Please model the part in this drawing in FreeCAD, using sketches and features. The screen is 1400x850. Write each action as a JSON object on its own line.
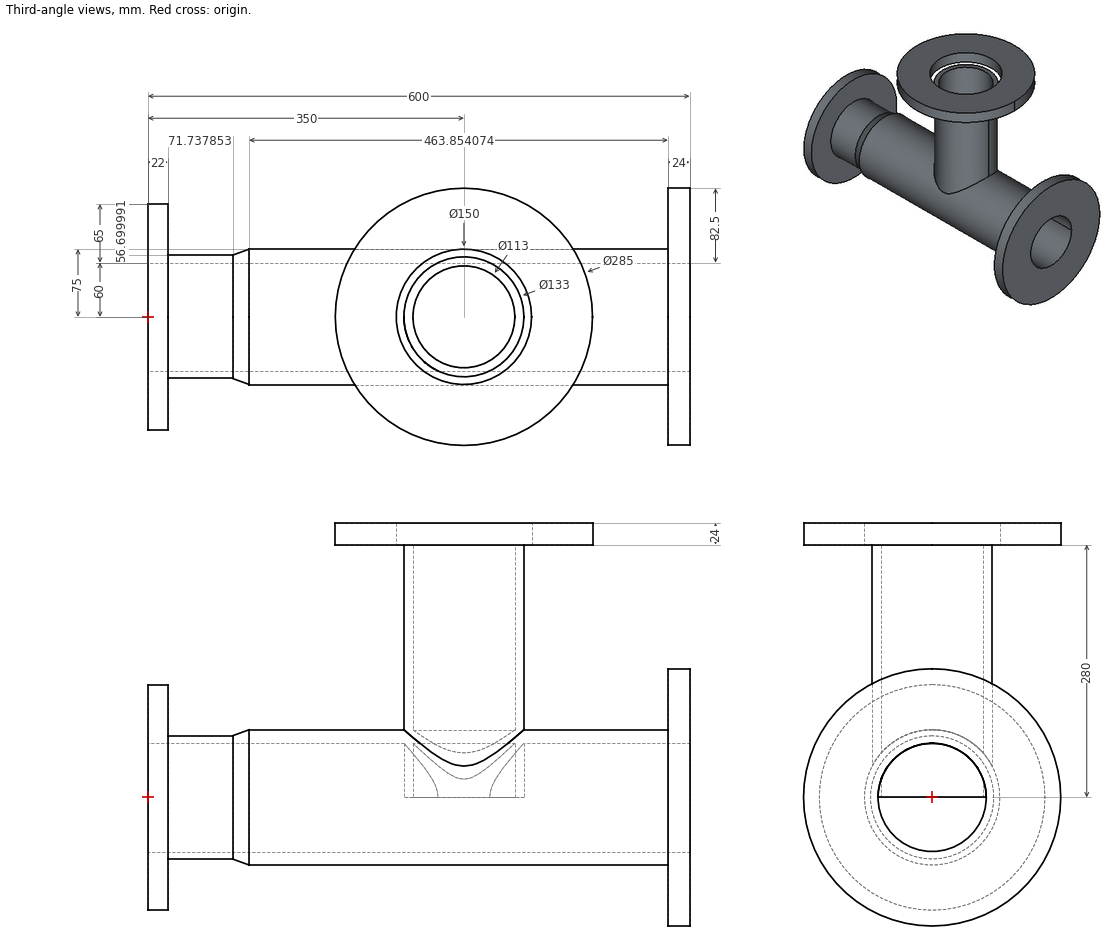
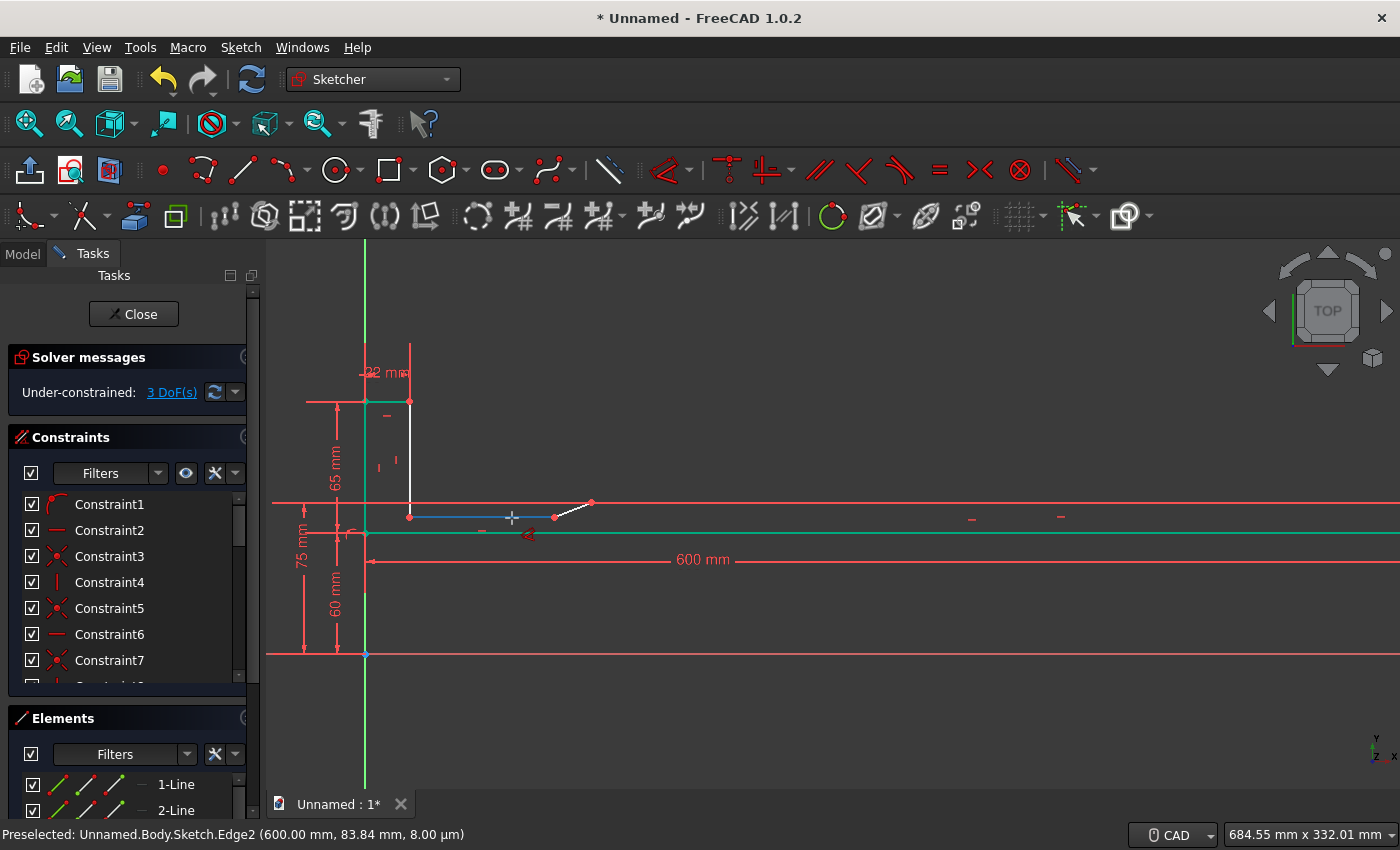
{"action": "left_click", "coordinate": [511, 517]}
{"action": "left_click", "coordinate": [482, 551]}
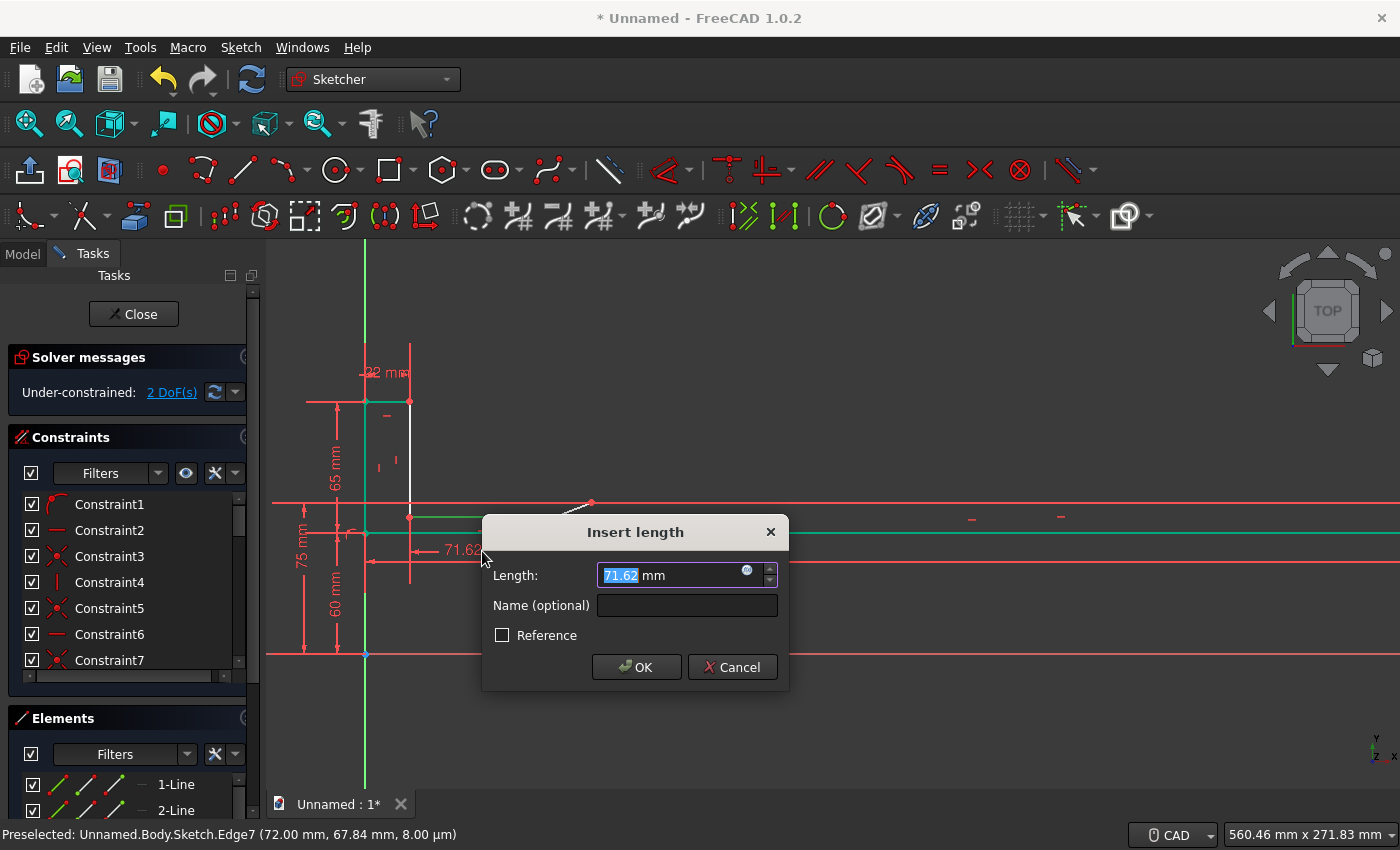
{"action": "type", "text": "71.737853"}
{"action": "key", "text": "Return"}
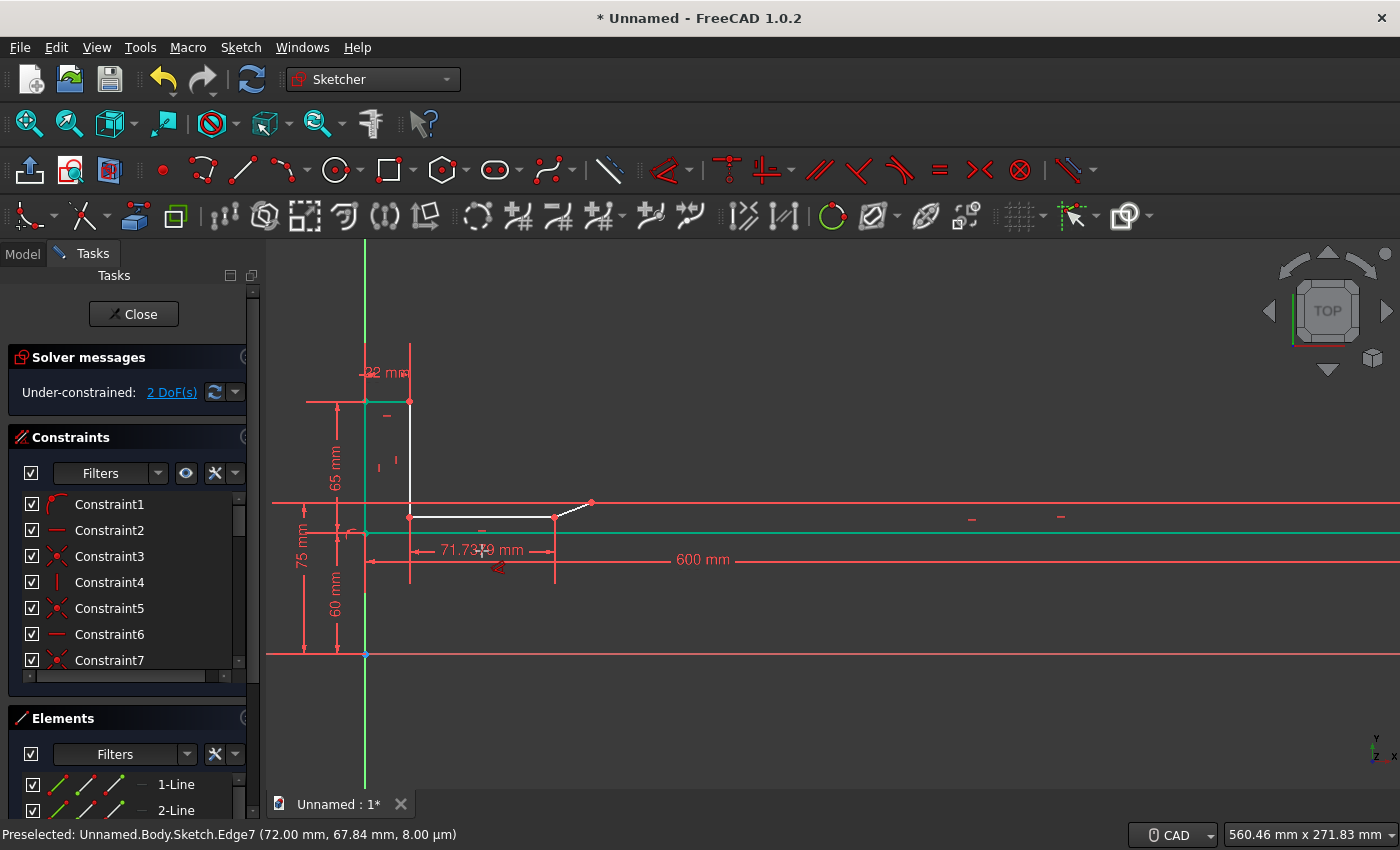
{"action": "left_click", "coordinate": [410, 482]}
{"action": "left_click", "coordinate": [444, 459]}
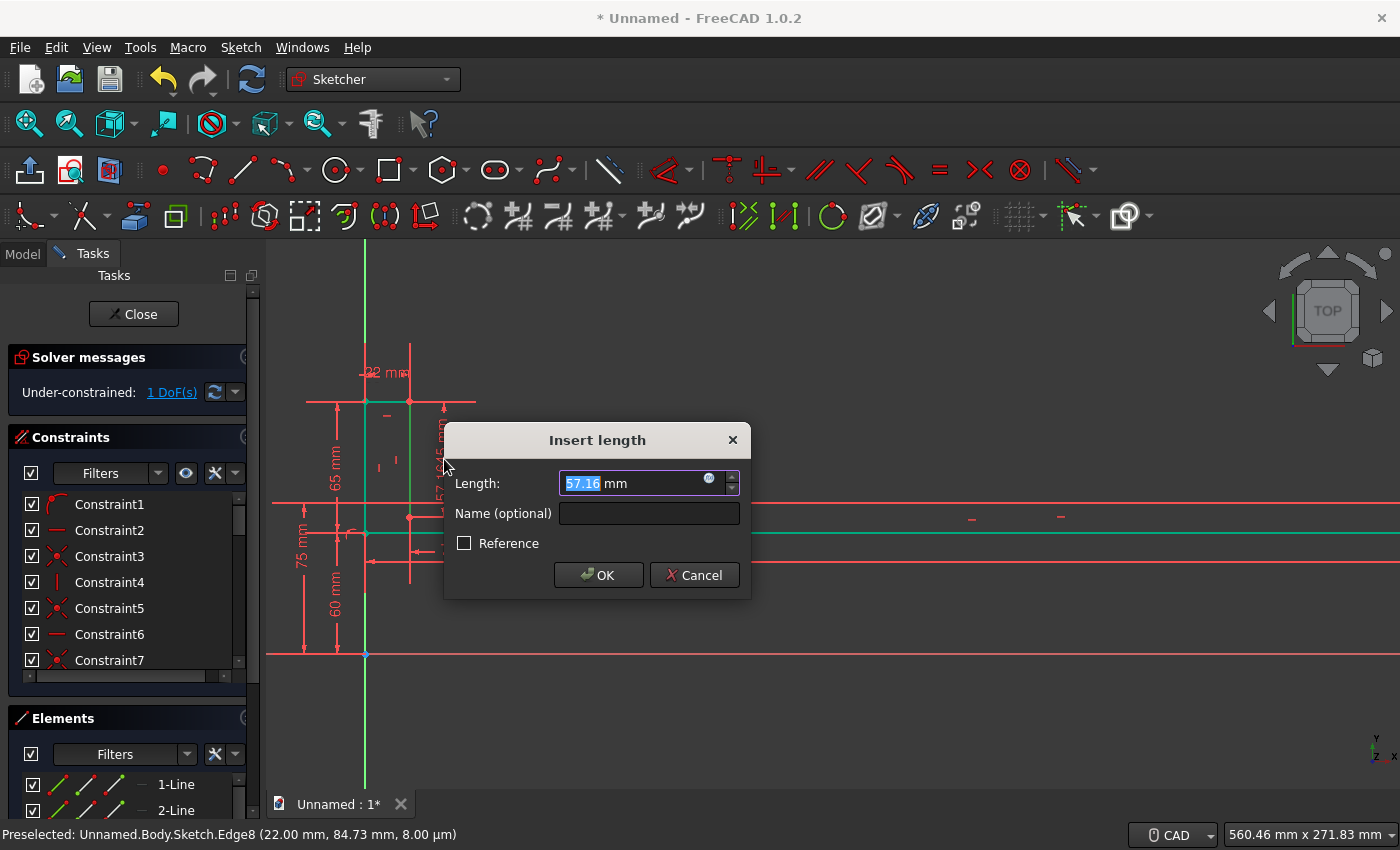
{"action": "type", "text": "56.699991"}
{"action": "key", "text": "Return"}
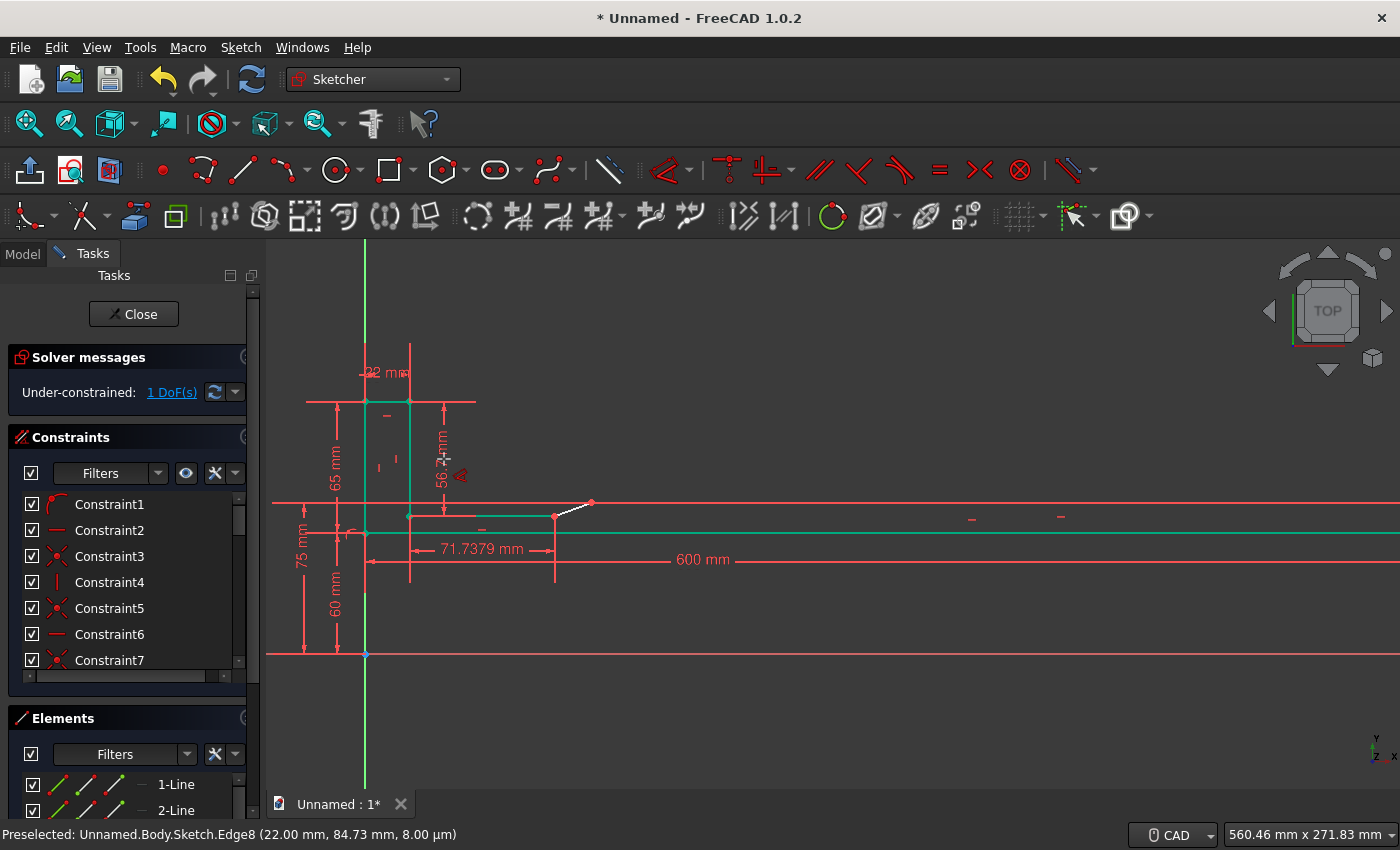
{"action": "left_click", "coordinate": [874, 503]}
{"action": "left_click", "coordinate": [913, 469]}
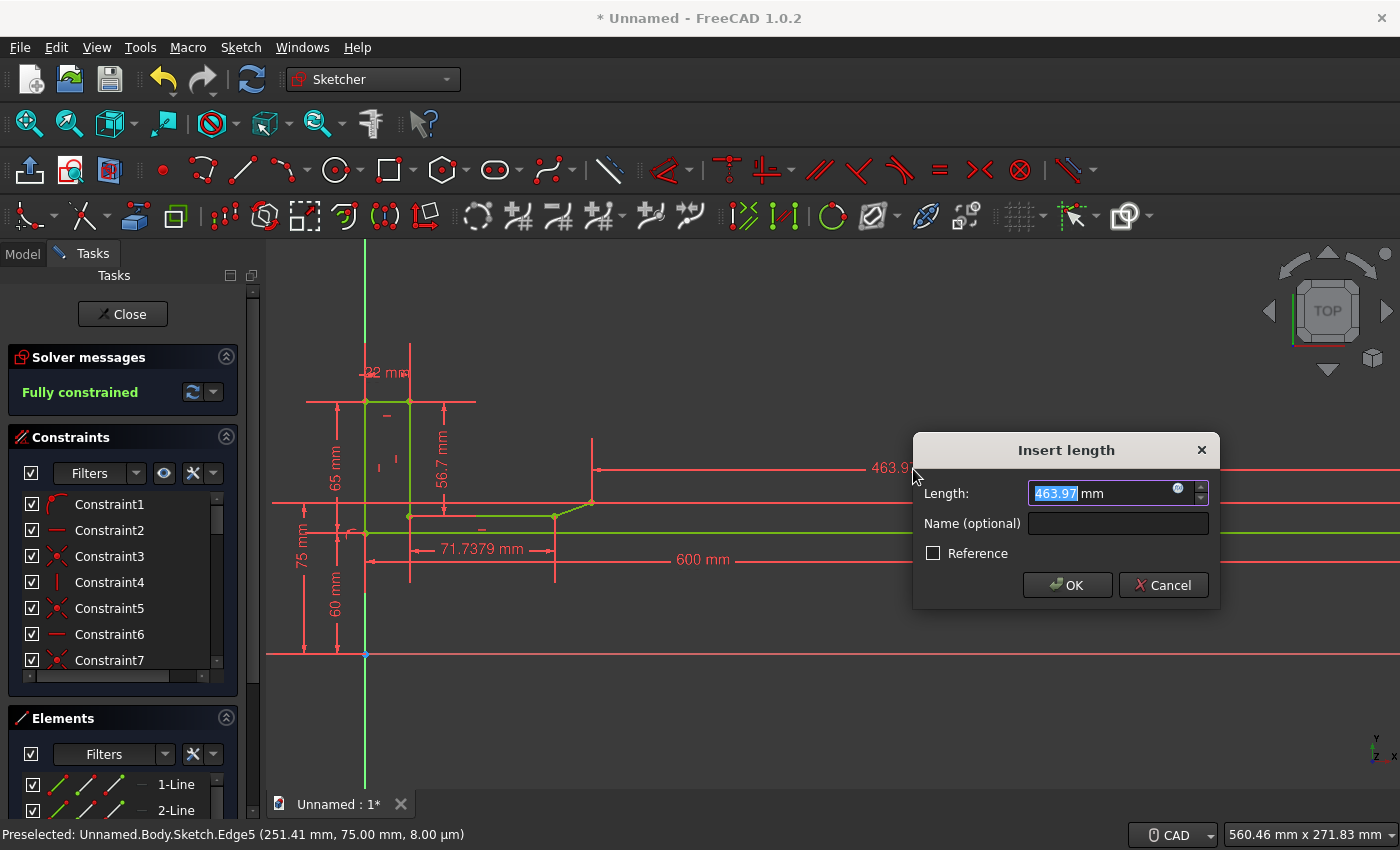
{"action": "type", "text": "463.854074"}
{"action": "key", "text": "Return"}
{"action": "key", "text": "Escape"}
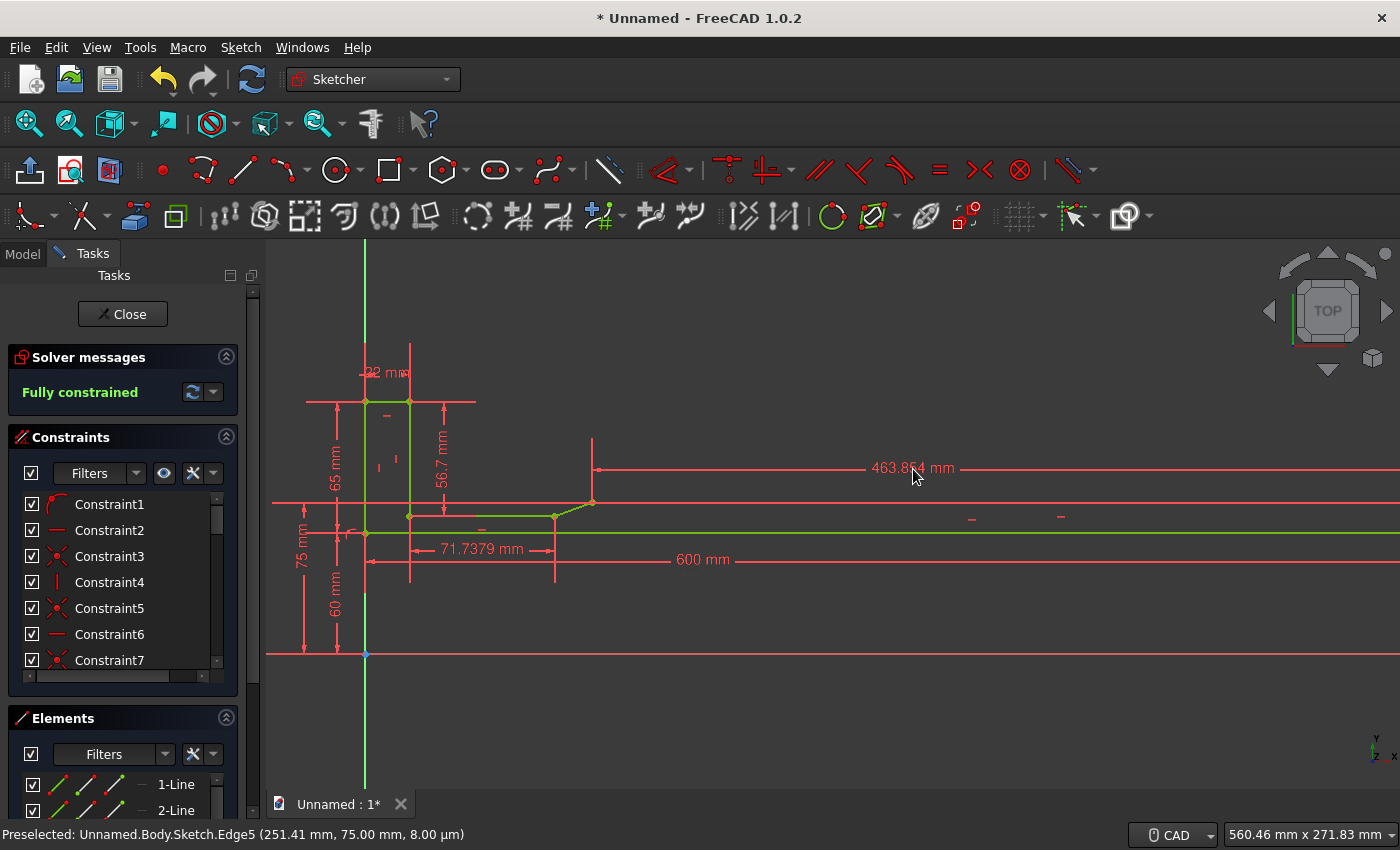
{"action": "left_click", "coordinate": [123, 314]}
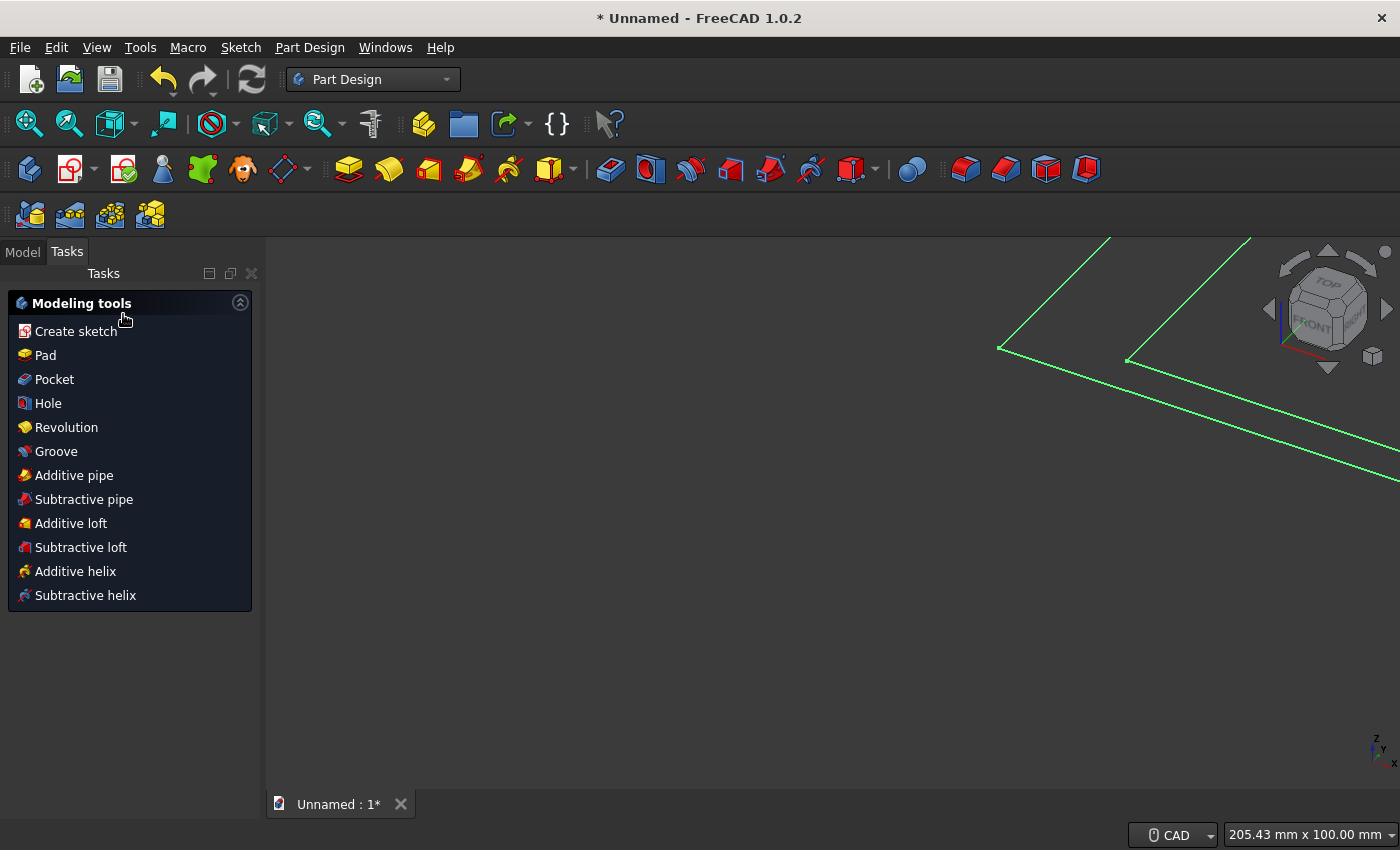
{"action": "left_click", "coordinate": [390, 170]}